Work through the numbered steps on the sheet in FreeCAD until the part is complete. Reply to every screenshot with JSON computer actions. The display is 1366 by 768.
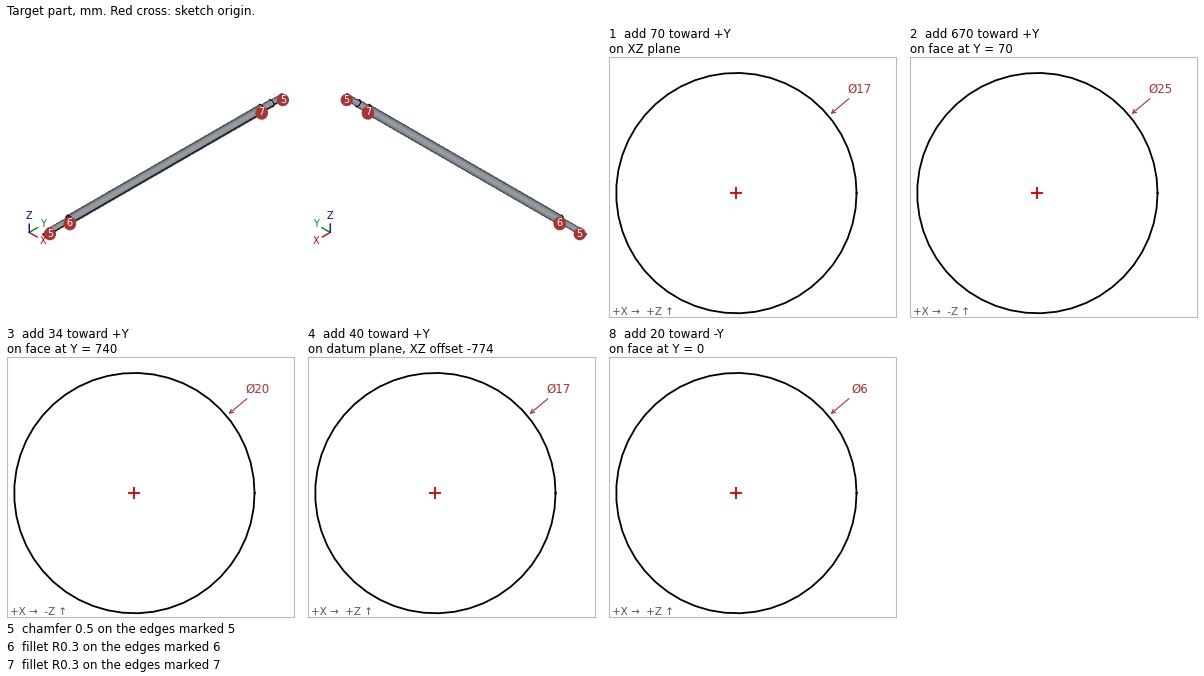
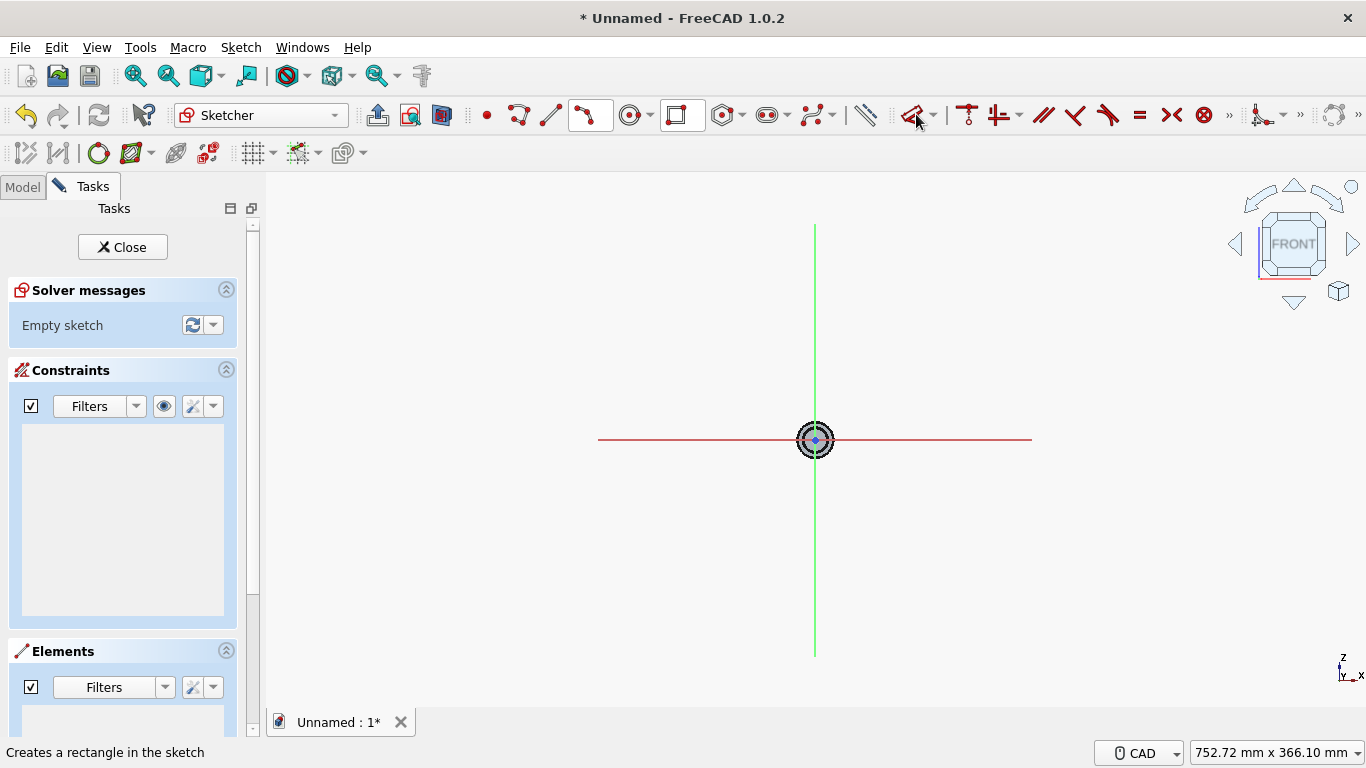
{"action": "scroll", "coordinate": [819, 440], "scroll_direction": "up", "scroll_amount": 15}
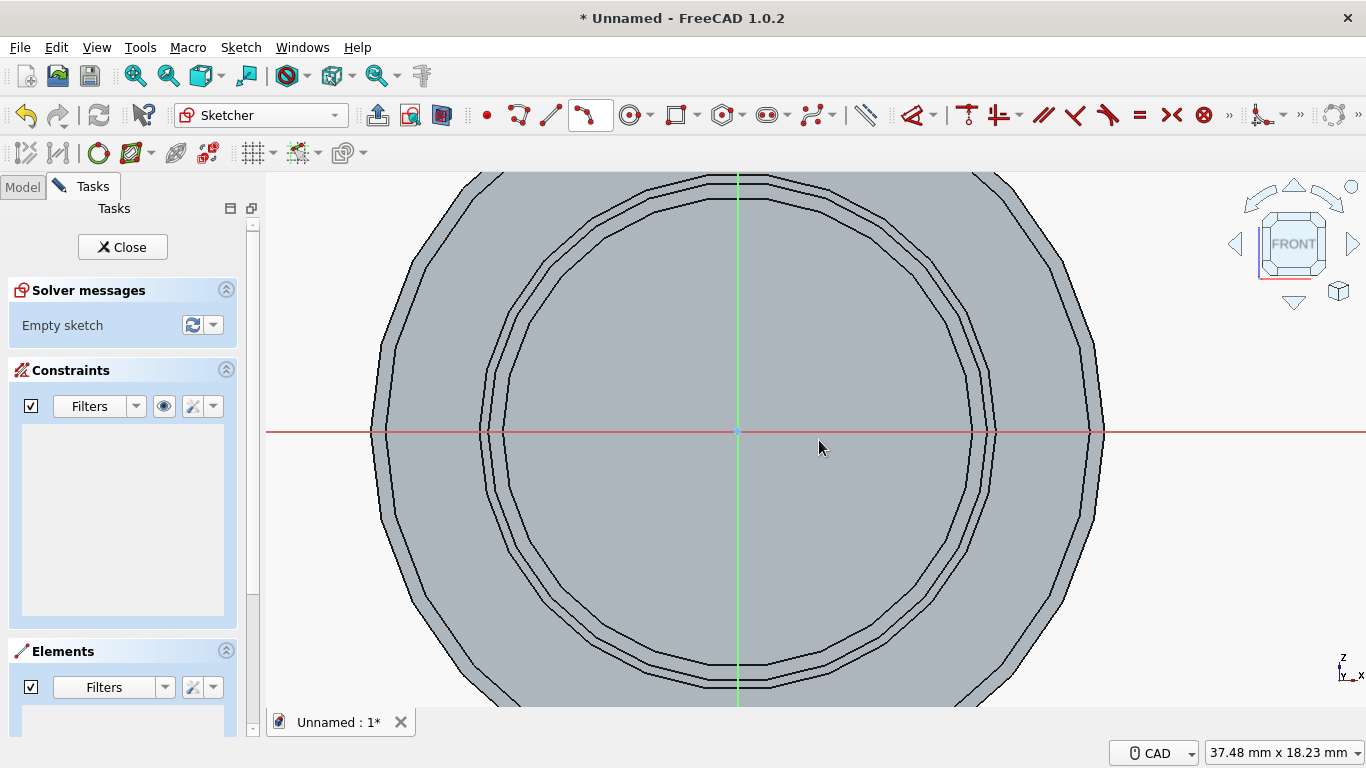
{"action": "scroll", "coordinate": [726, 423], "scroll_direction": "up", "scroll_amount": 3}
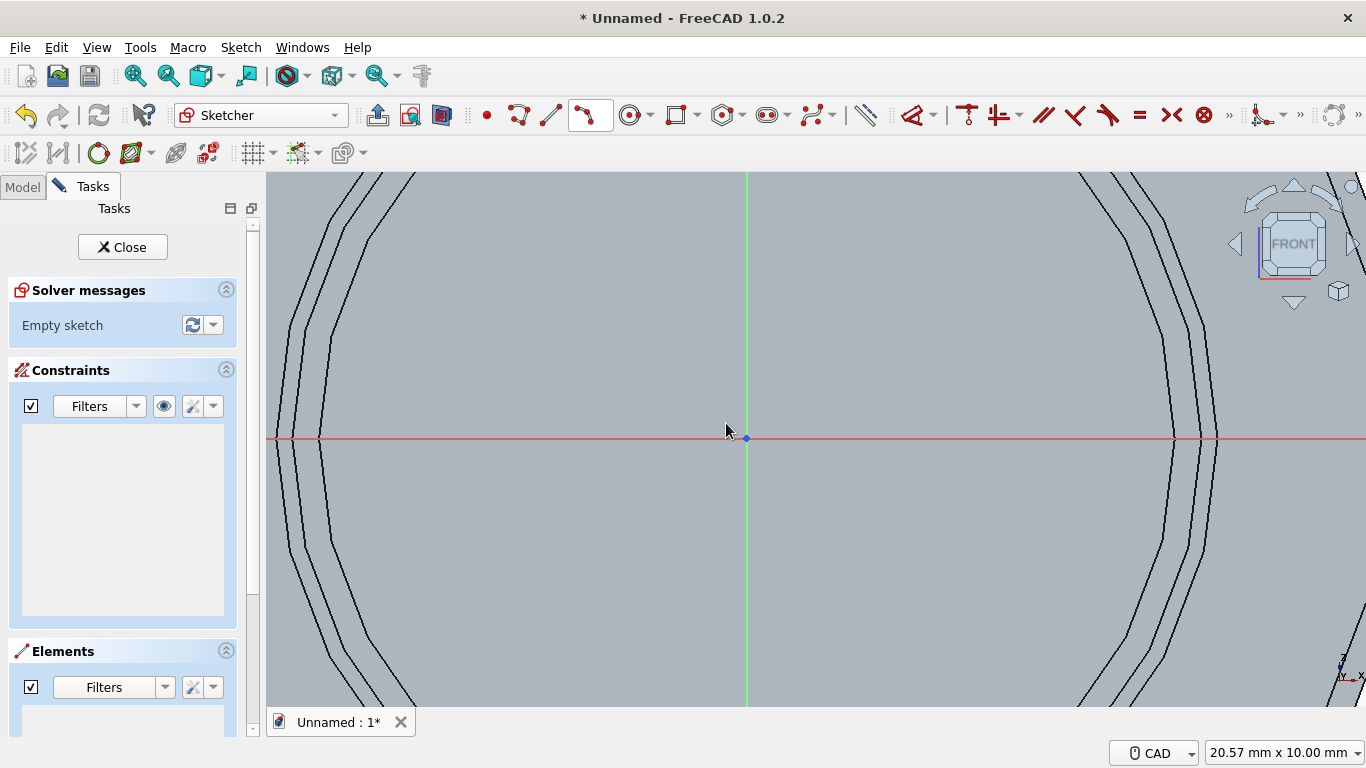
{"action": "key", "text": "g c"}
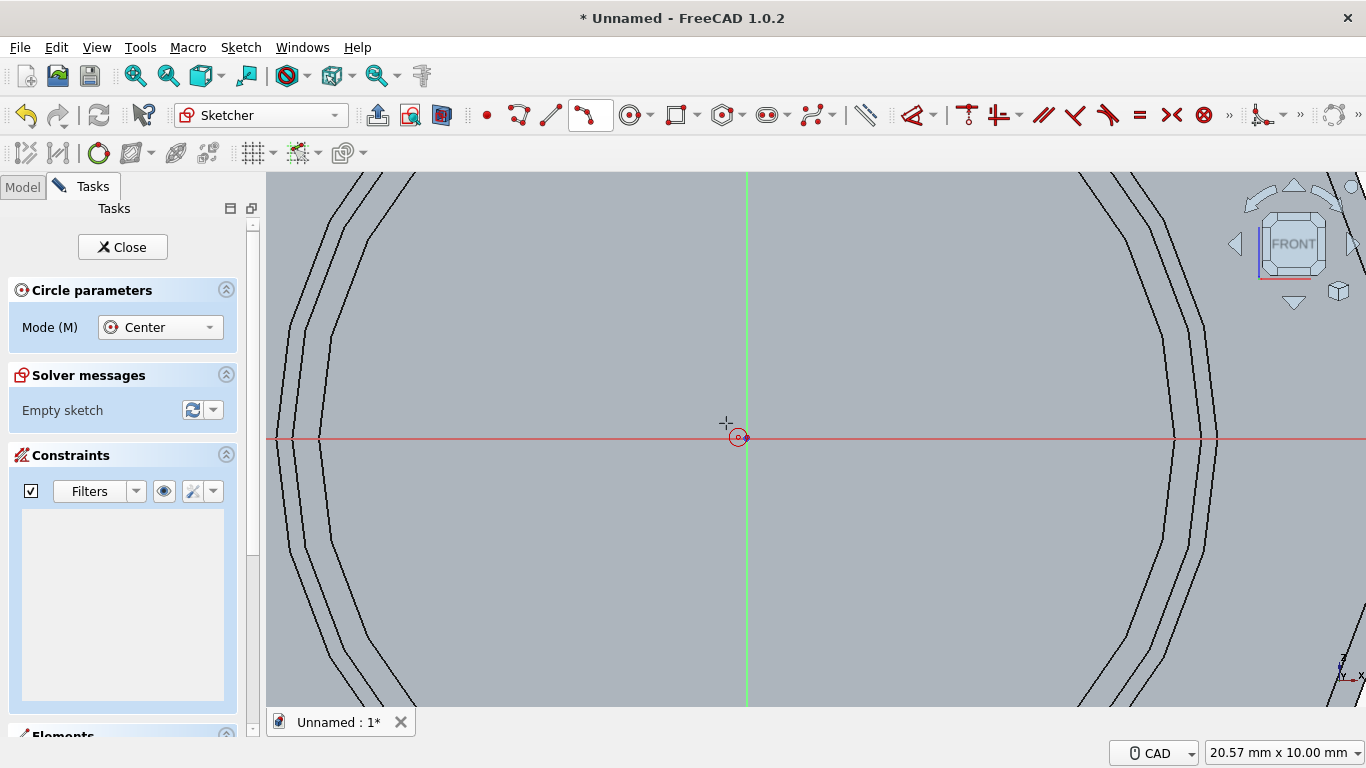
{"action": "left_click", "coordinate": [747, 439]}
{"action": "left_click", "coordinate": [860, 325]}
{"action": "key", "text": "Escape"}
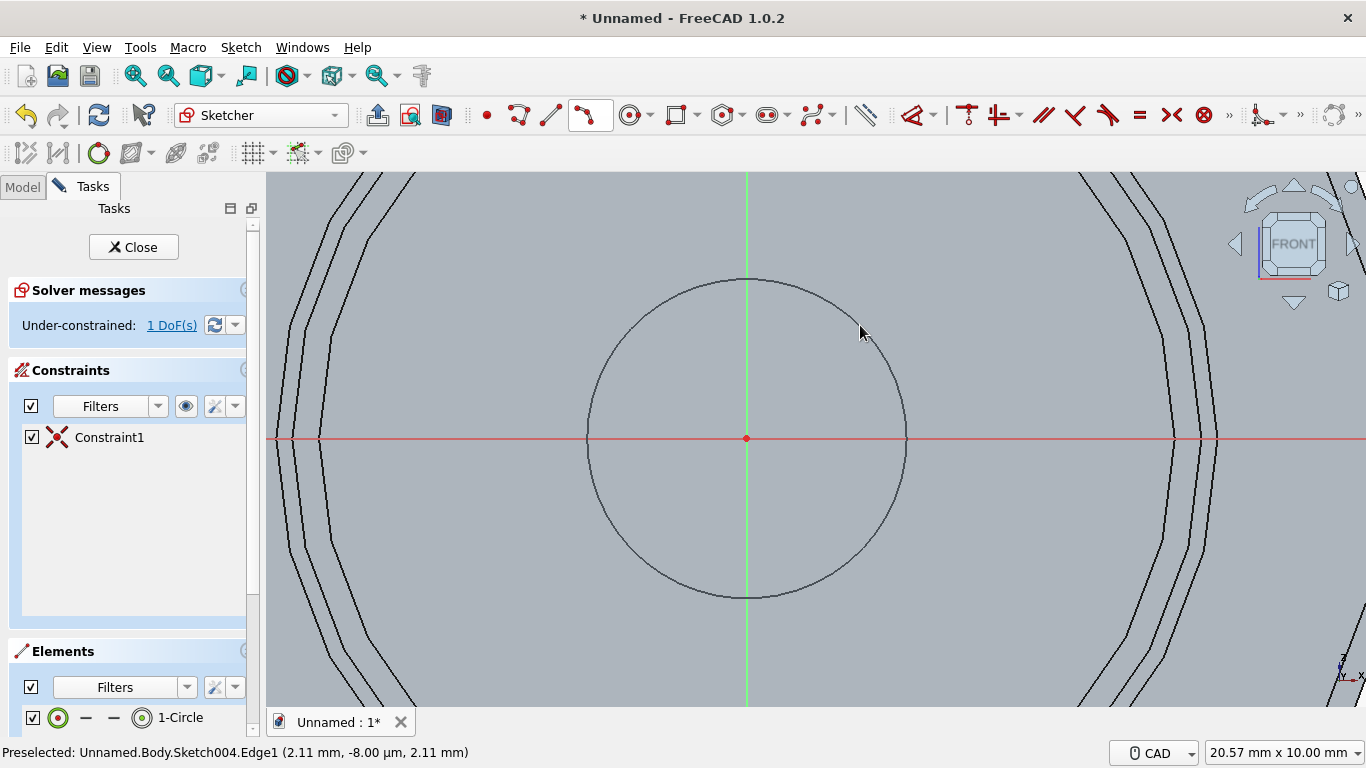
{"action": "key", "text": "d"}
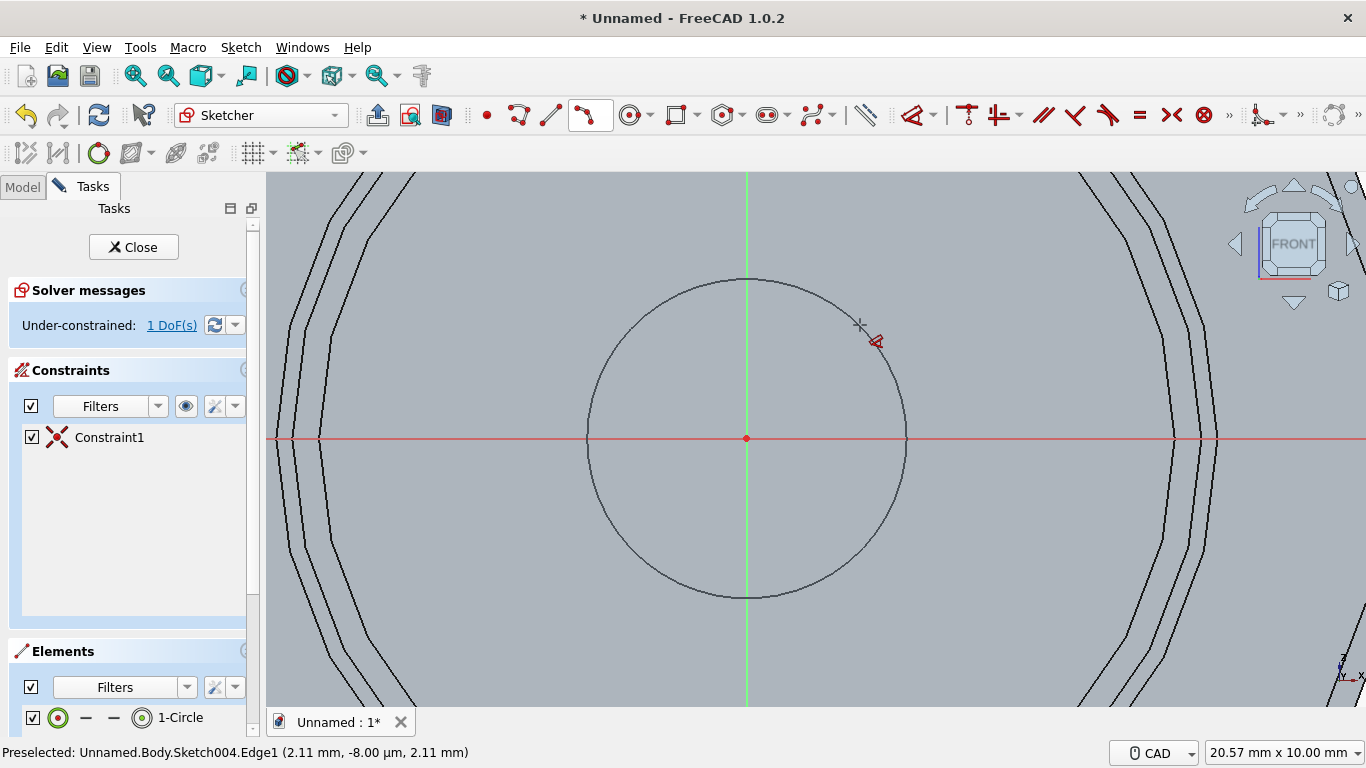
{"action": "left_click", "coordinate": [859, 325]}
{"action": "left_click", "coordinate": [881, 302]}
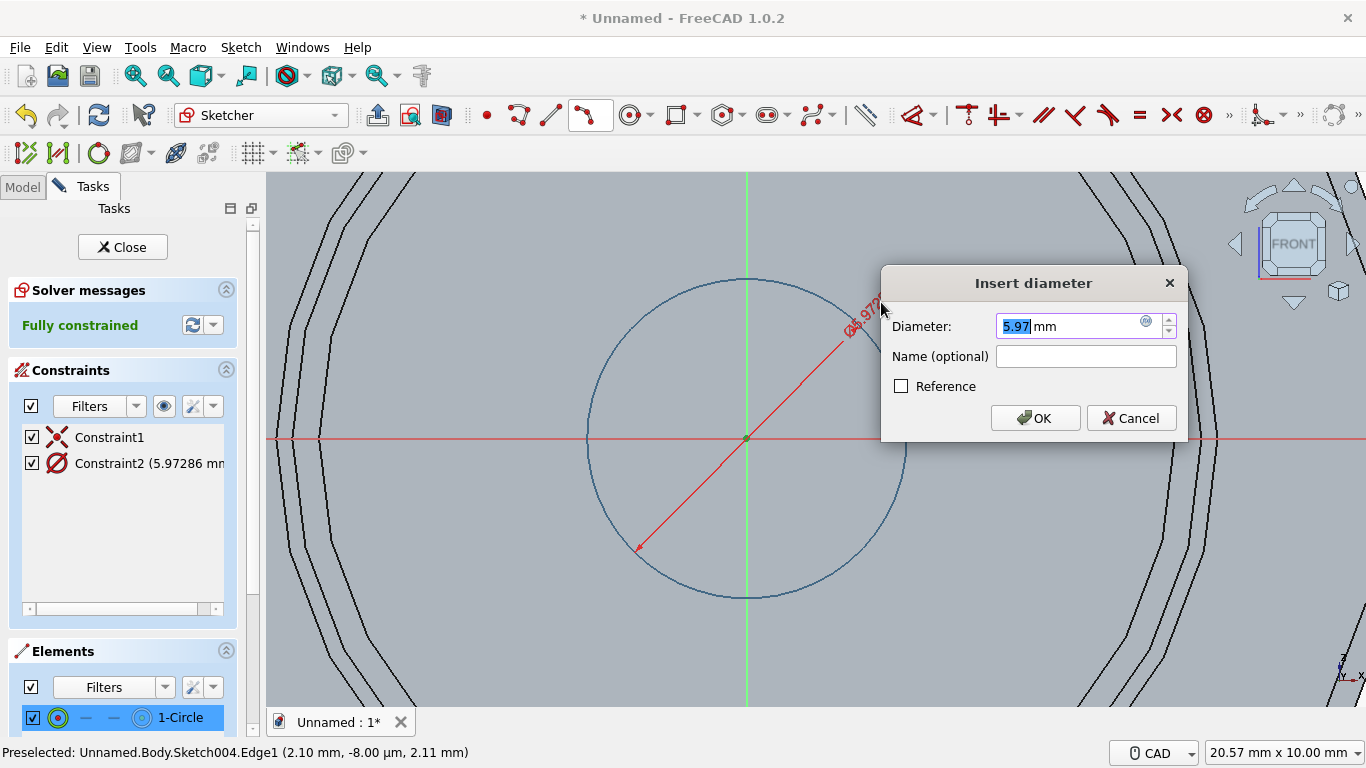
{"action": "type", "text": "6"}
{"action": "key", "text": "Return"}
{"action": "key", "text": "Escape"}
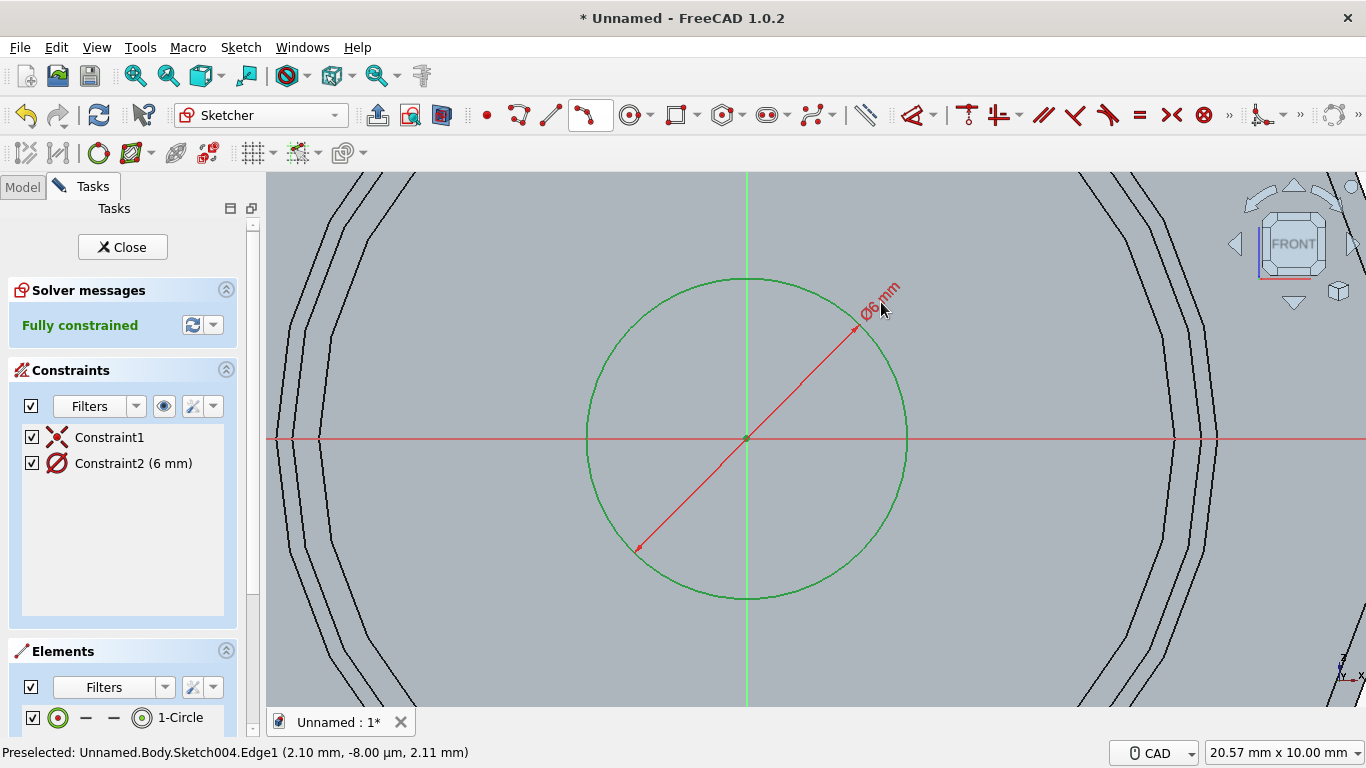
{"action": "left_click", "coordinate": [123, 247]}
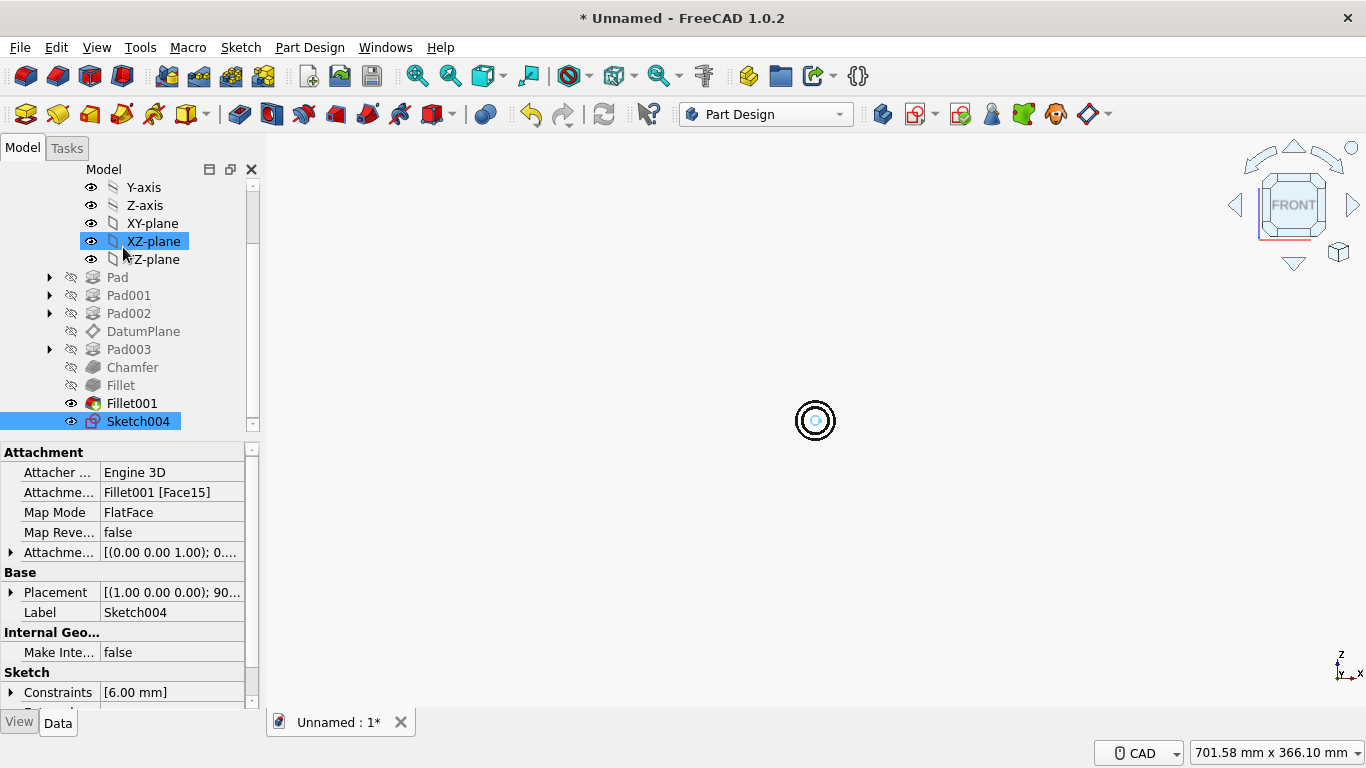
{"action": "left_click", "coordinate": [26, 114]}